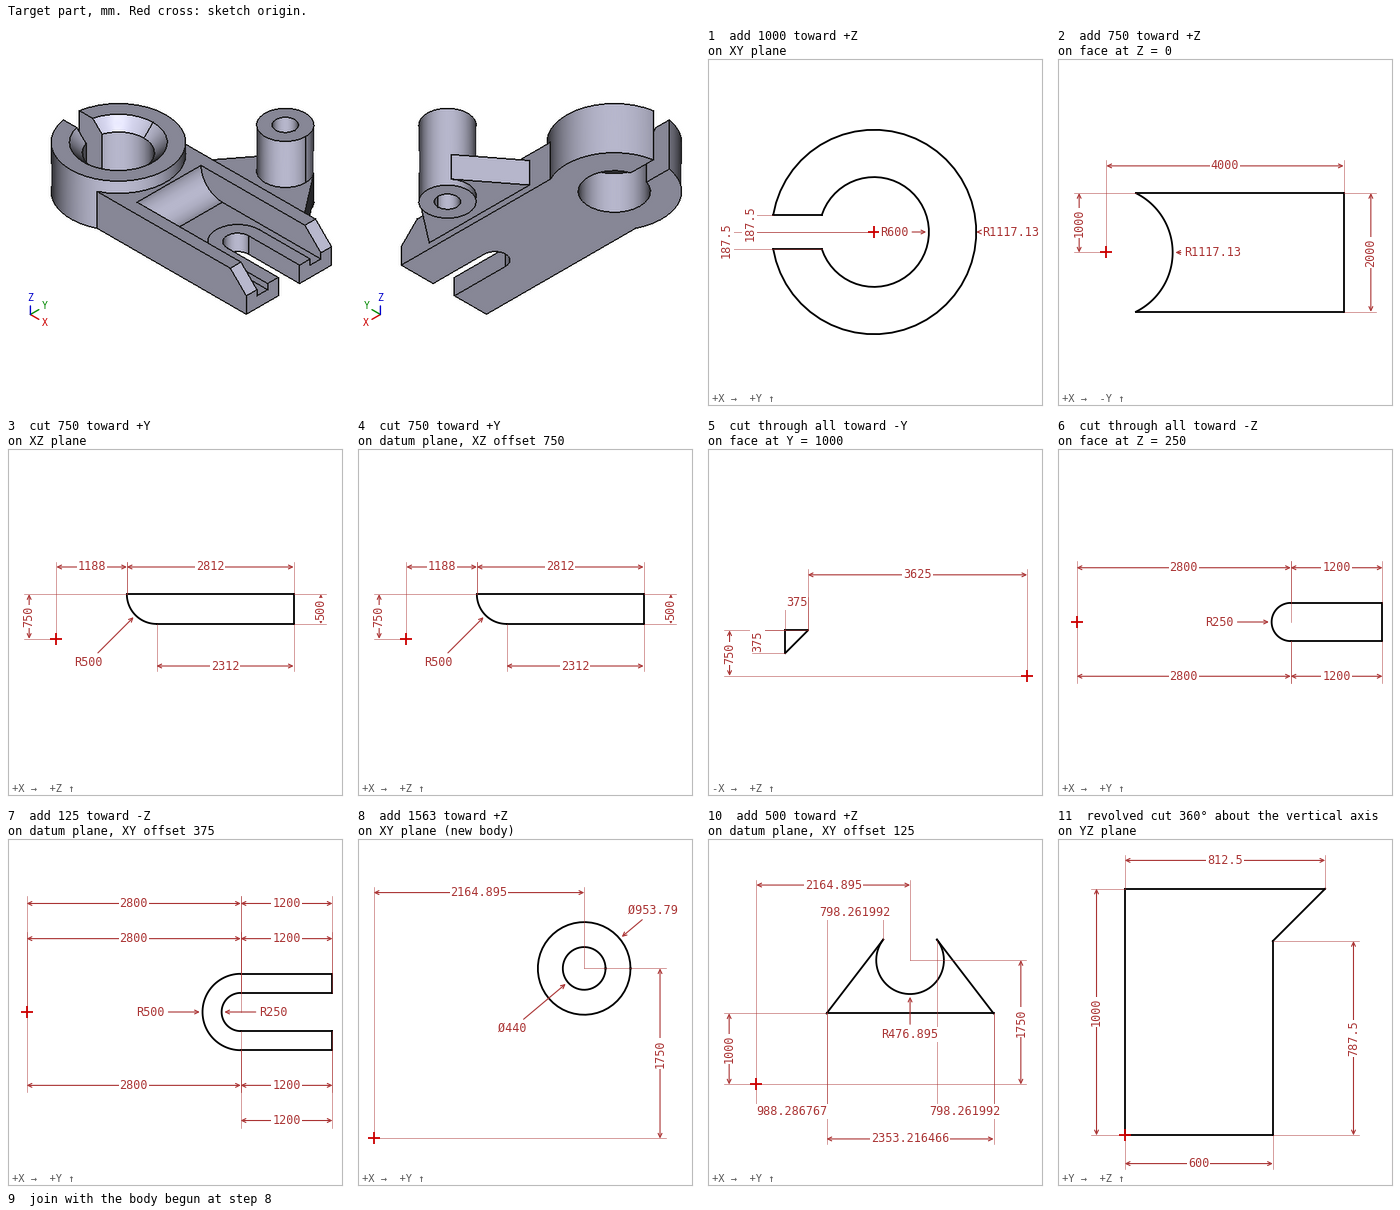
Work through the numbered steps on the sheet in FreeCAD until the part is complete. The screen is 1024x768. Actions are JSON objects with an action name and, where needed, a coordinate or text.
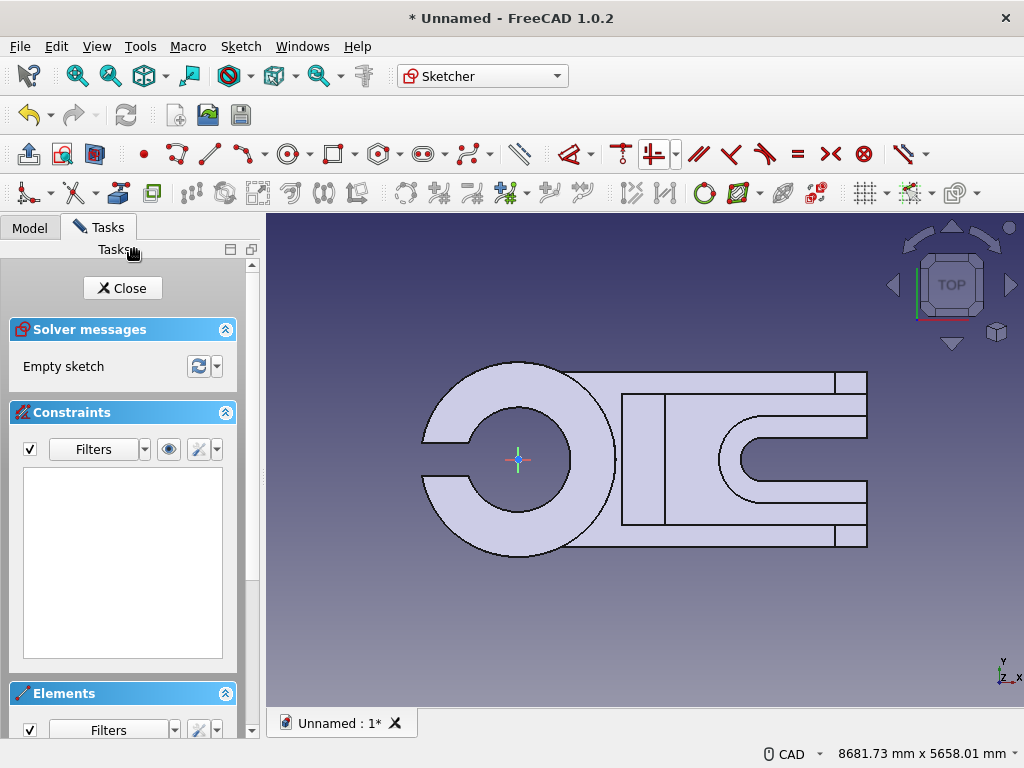
{"action": "scroll", "coordinate": [750, 257], "scroll_direction": "up", "scroll_amount": 7}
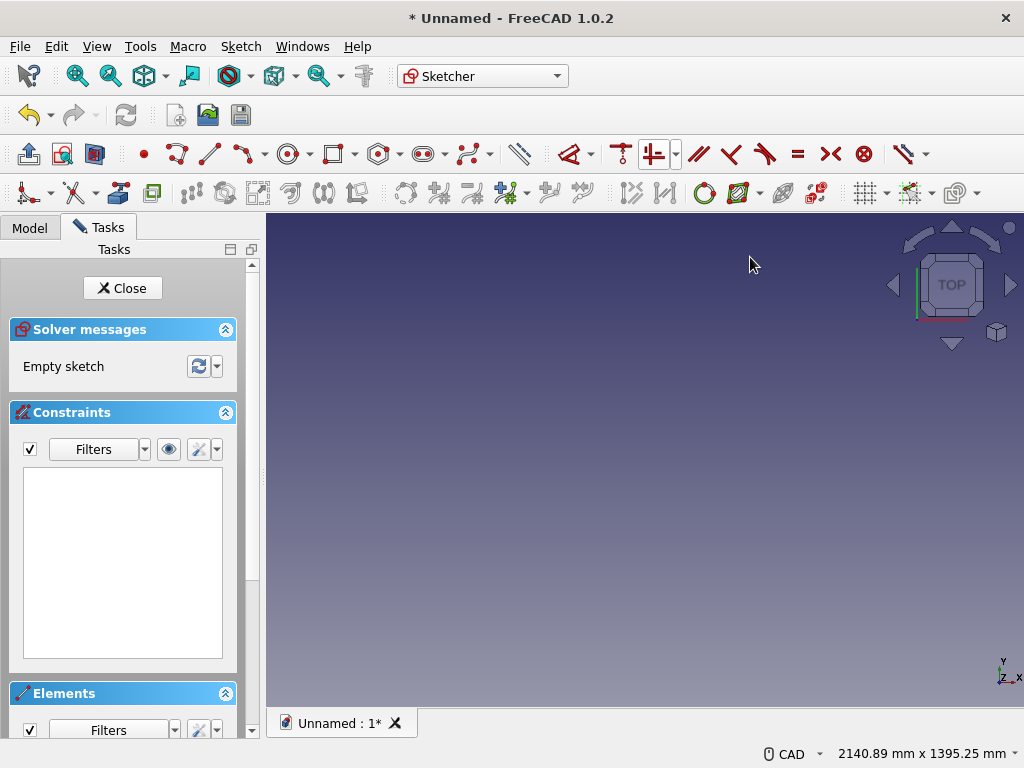
{"action": "key", "text": "g c"}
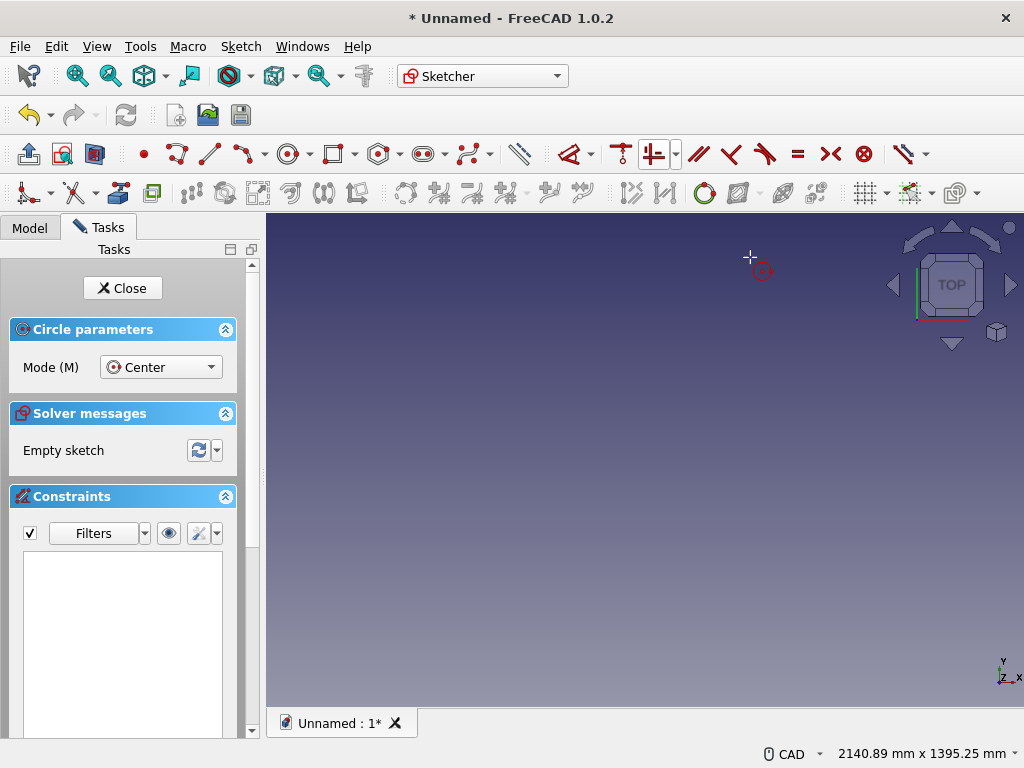
{"action": "left_click", "coordinate": [574, 459]}
{"action": "mouse_move", "coordinate": [693, 339]}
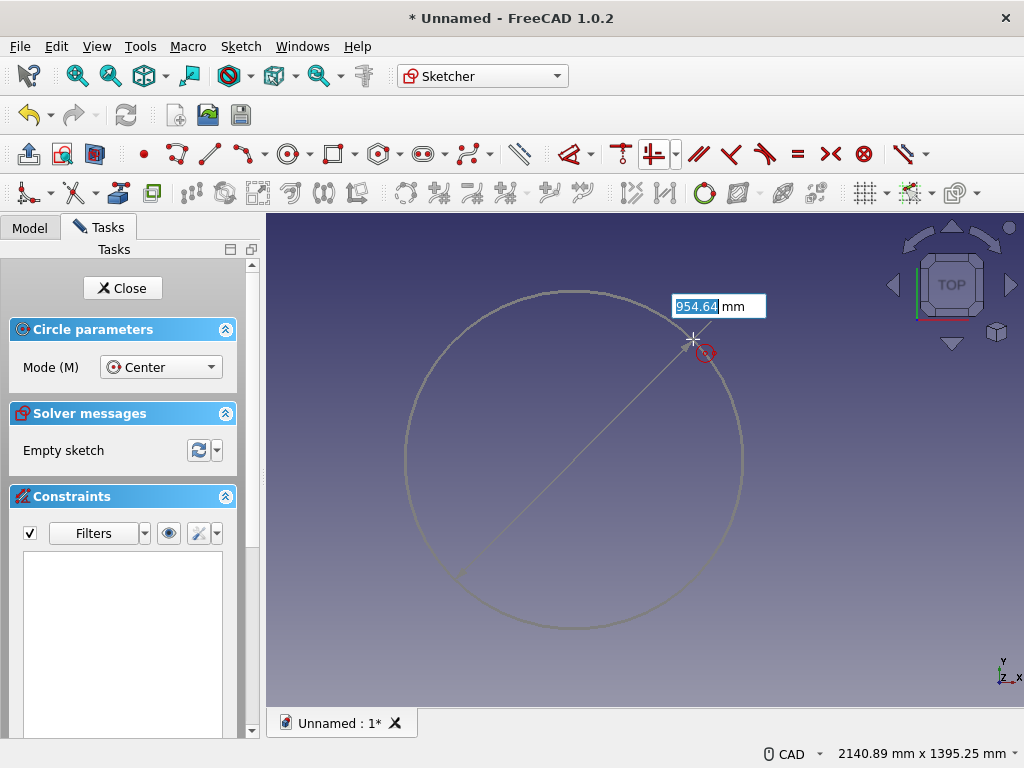
{"action": "type", "text": "953.79"}
{"action": "key", "text": "Return"}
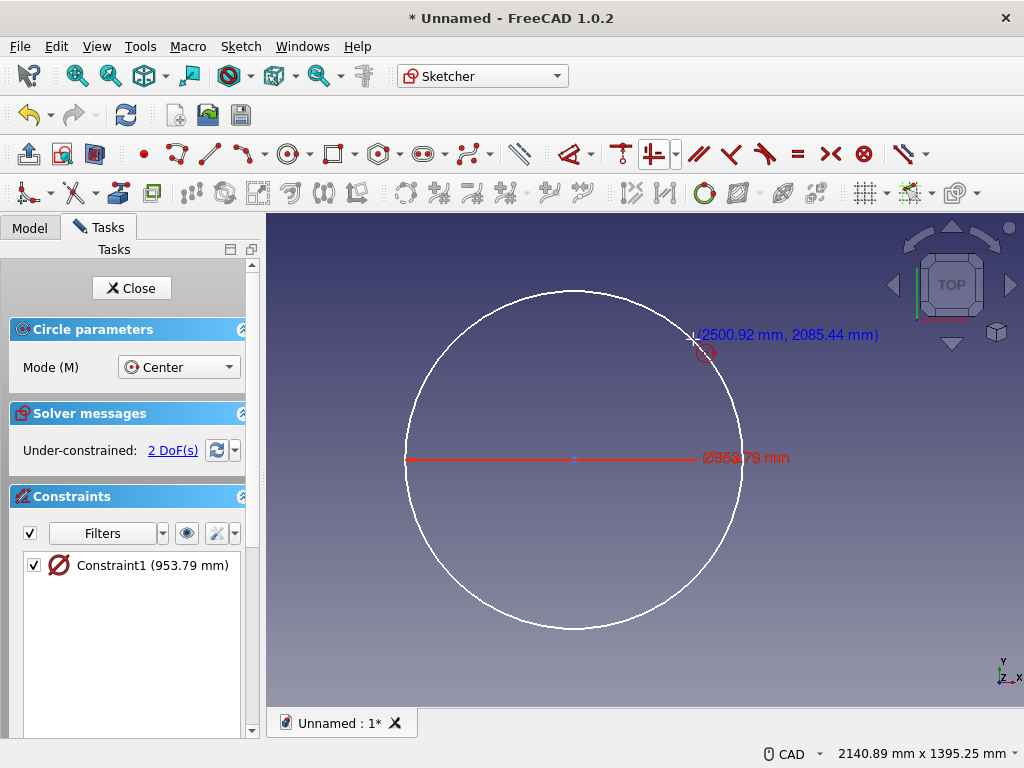
{"action": "left_click", "coordinate": [574, 460]}
{"action": "mouse_move", "coordinate": [629, 404]}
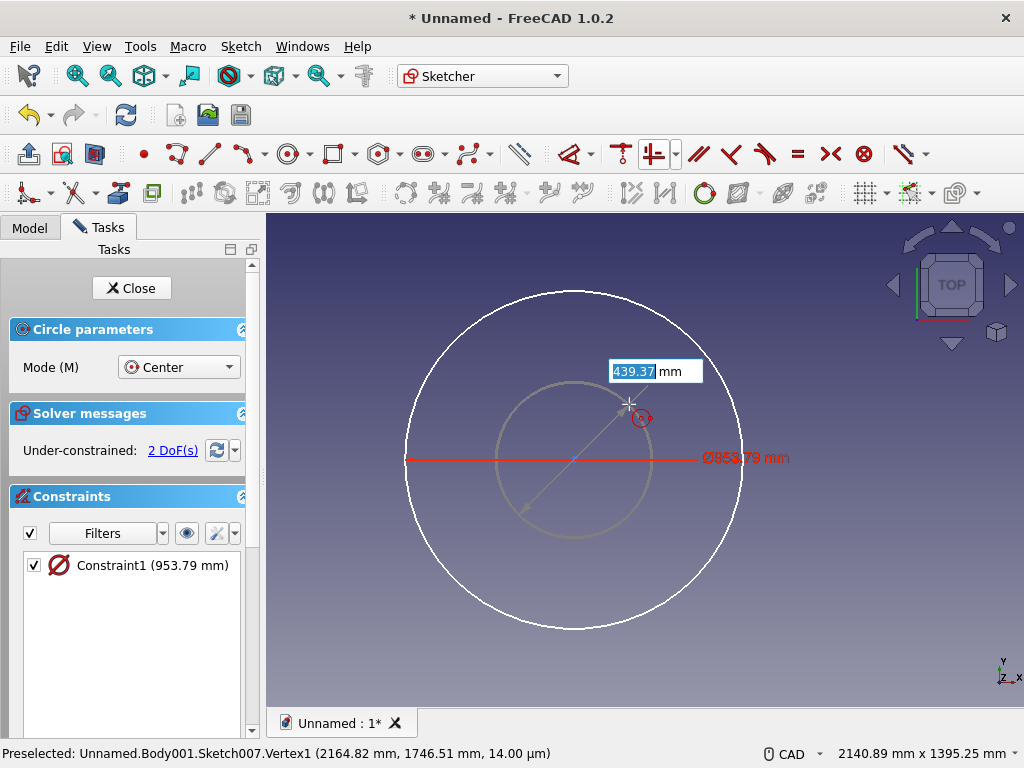
{"action": "type", "text": "440"}
{"action": "key", "text": "Return"}
{"action": "key", "text": "Escape"}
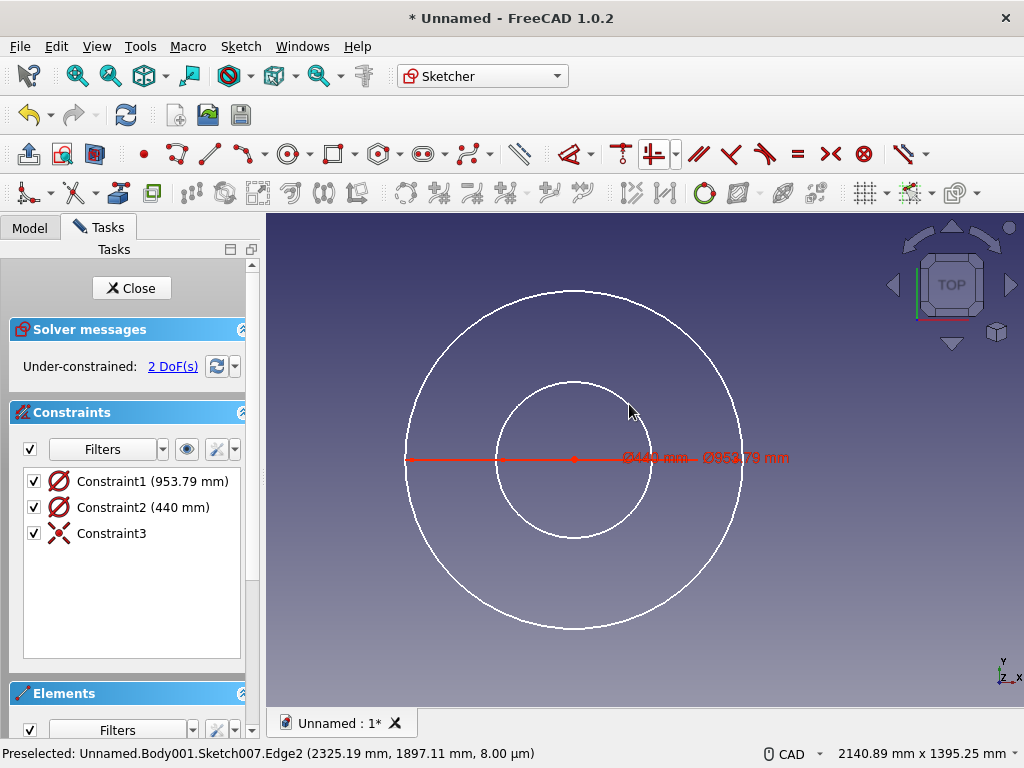
{"action": "key", "text": "d"}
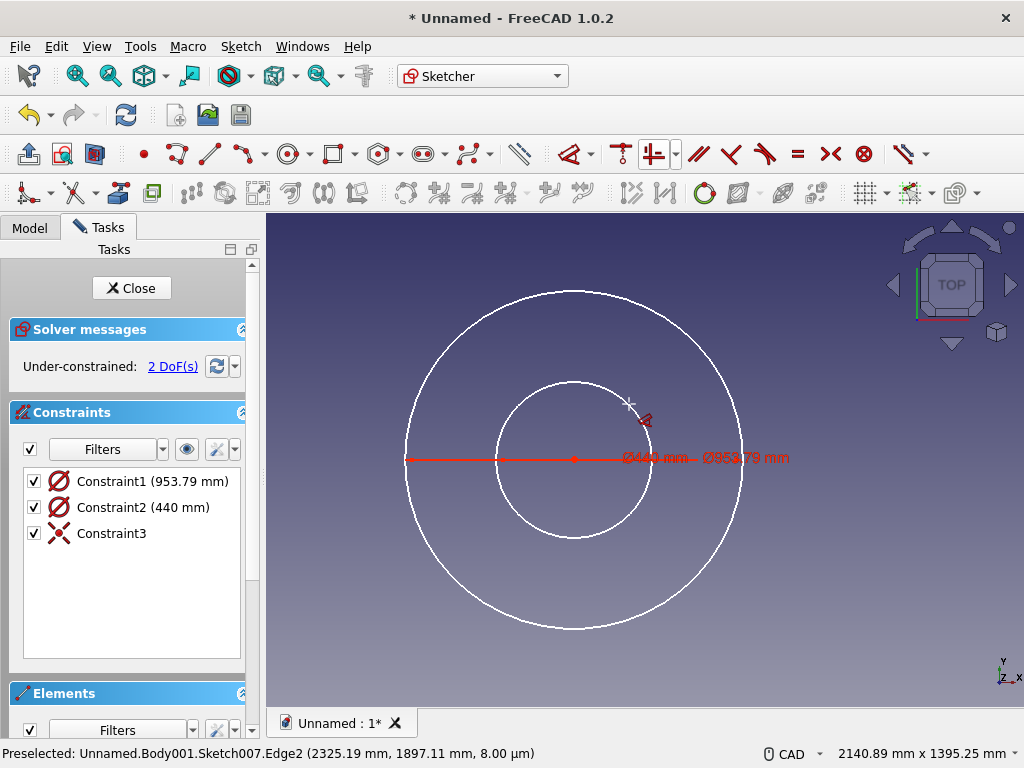
{"action": "left_click", "coordinate": [574, 460]}
{"action": "left_click", "coordinate": [608, 570]}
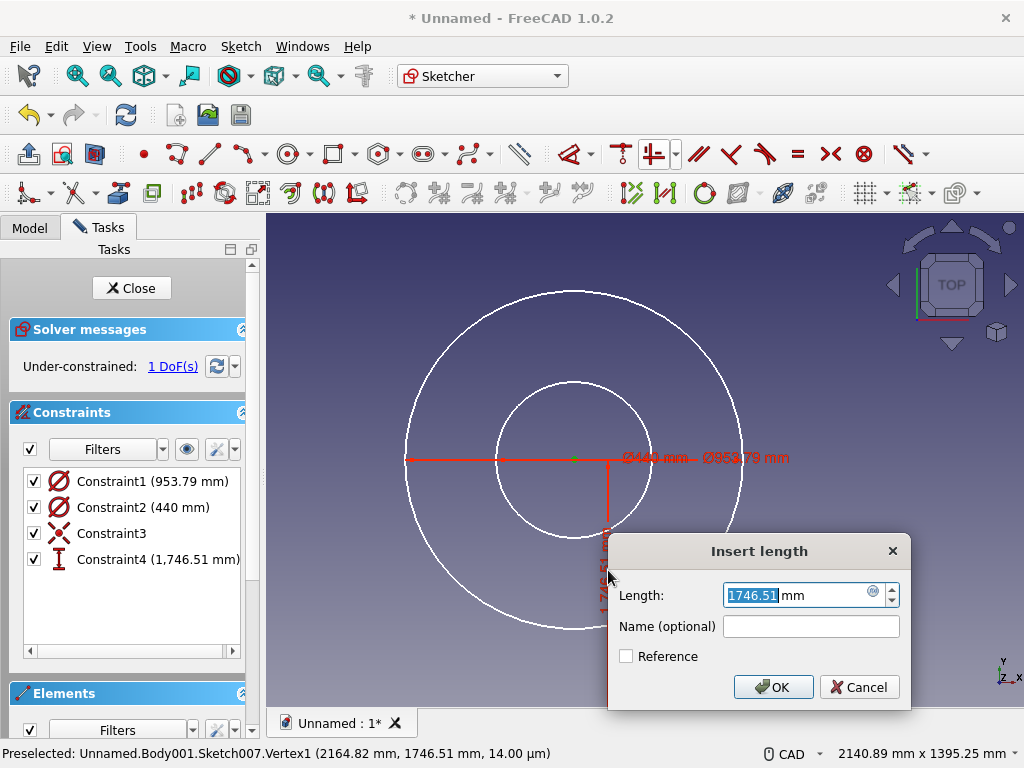
{"action": "type", "text": "1750"}
{"action": "key", "text": "Return"}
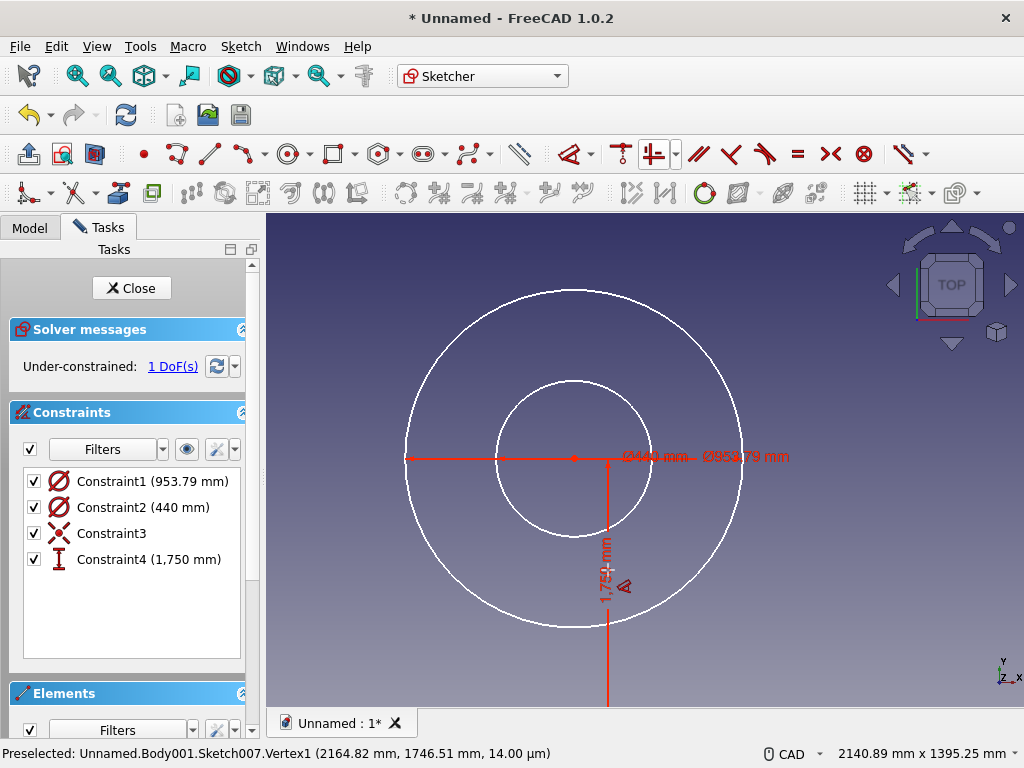
{"action": "left_click", "coordinate": [574, 459]}
{"action": "left_click", "coordinate": [434, 425]}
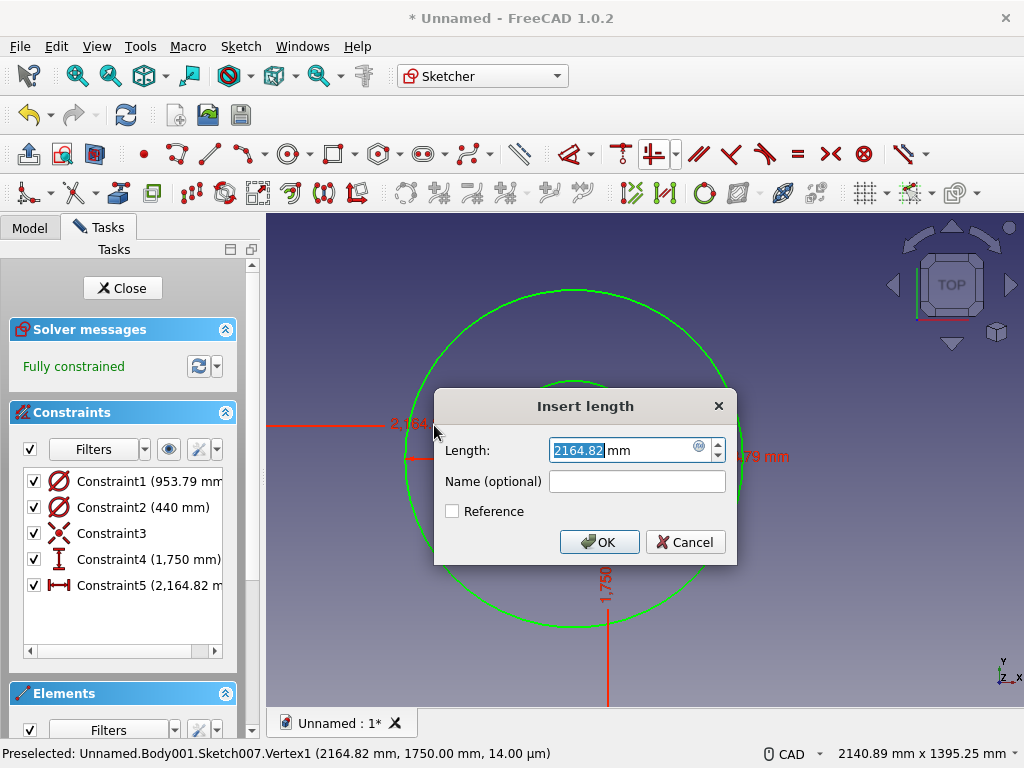
{"action": "type", "text": "2164.895"}
{"action": "key", "text": "Return"}
{"action": "key", "text": "Escape"}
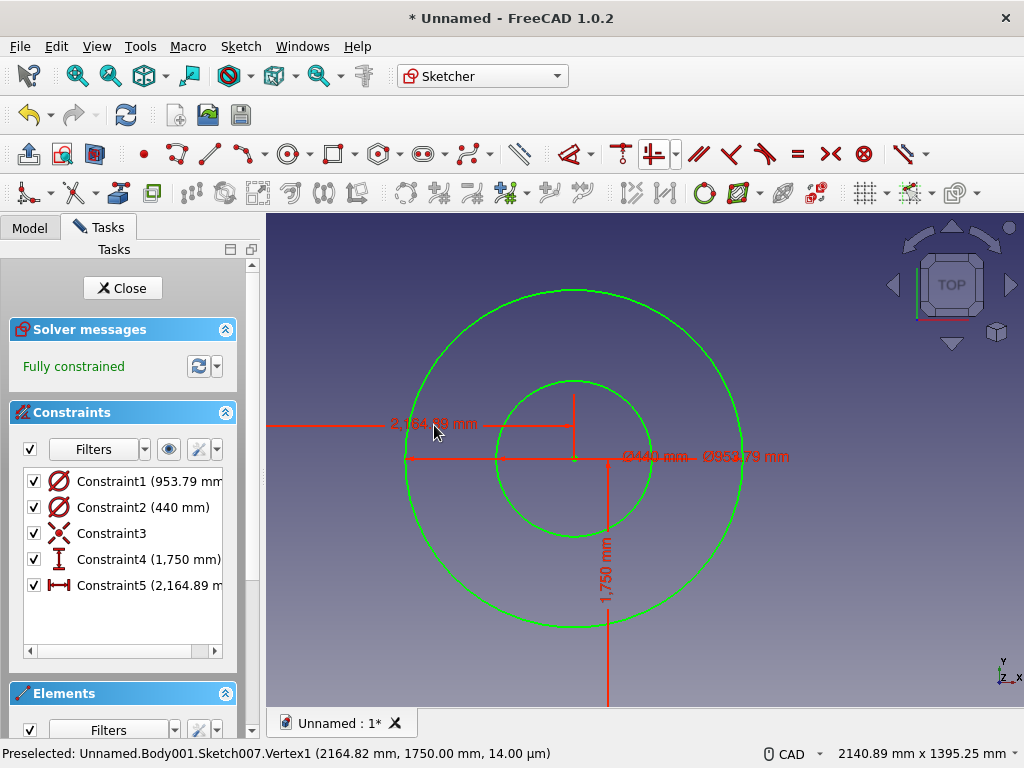
{"action": "left_click", "coordinate": [123, 288]}